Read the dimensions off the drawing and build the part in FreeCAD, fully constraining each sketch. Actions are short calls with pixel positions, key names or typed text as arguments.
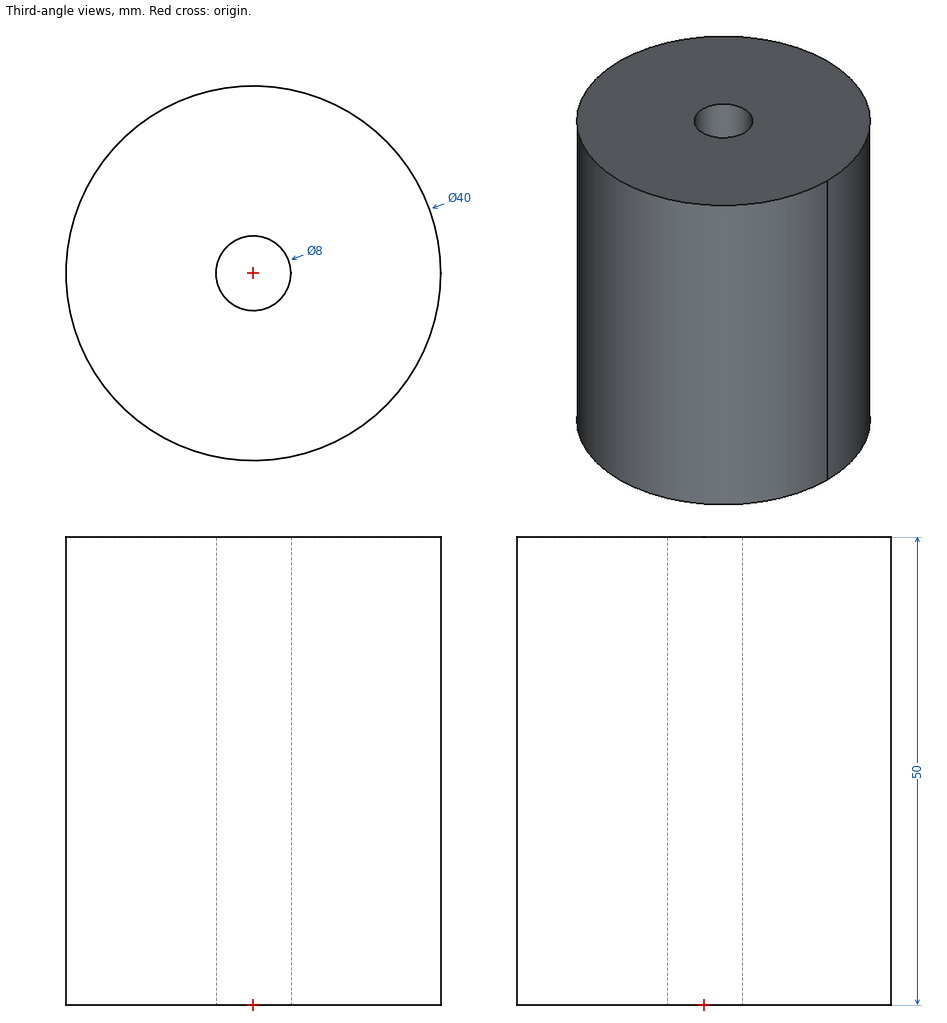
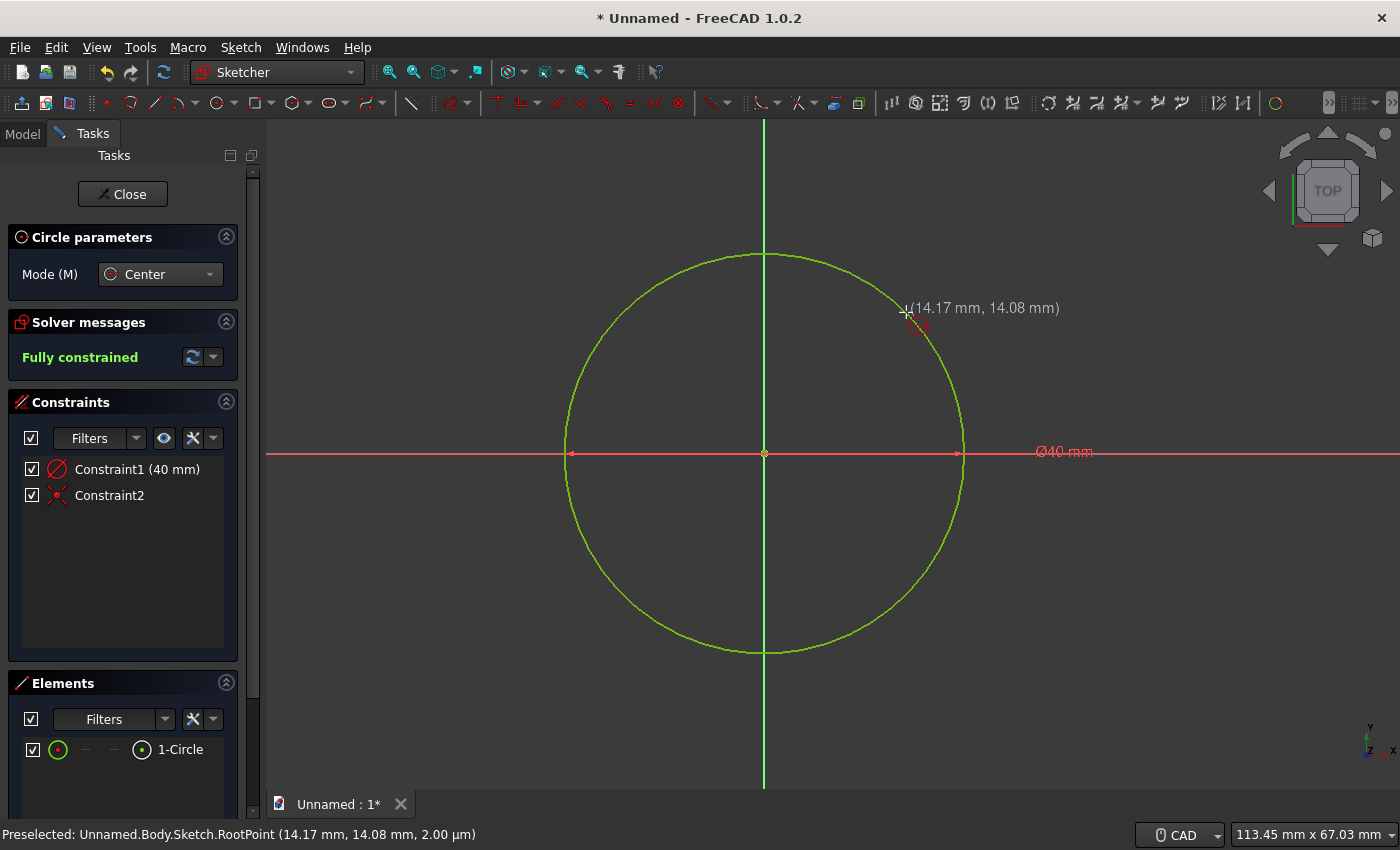
click(764, 454)
move(793, 425)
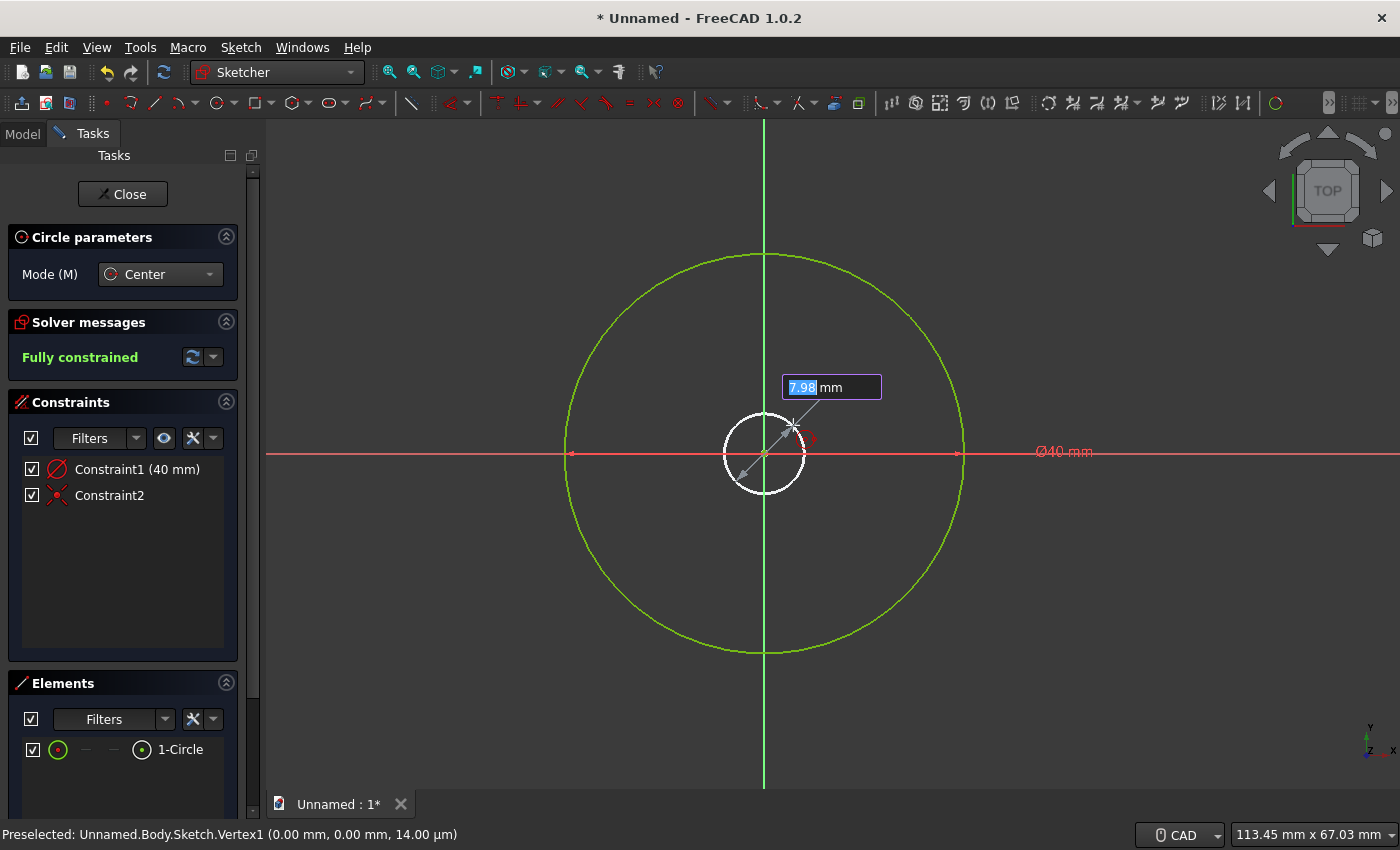
text(8)
key(Return)
key(Escape)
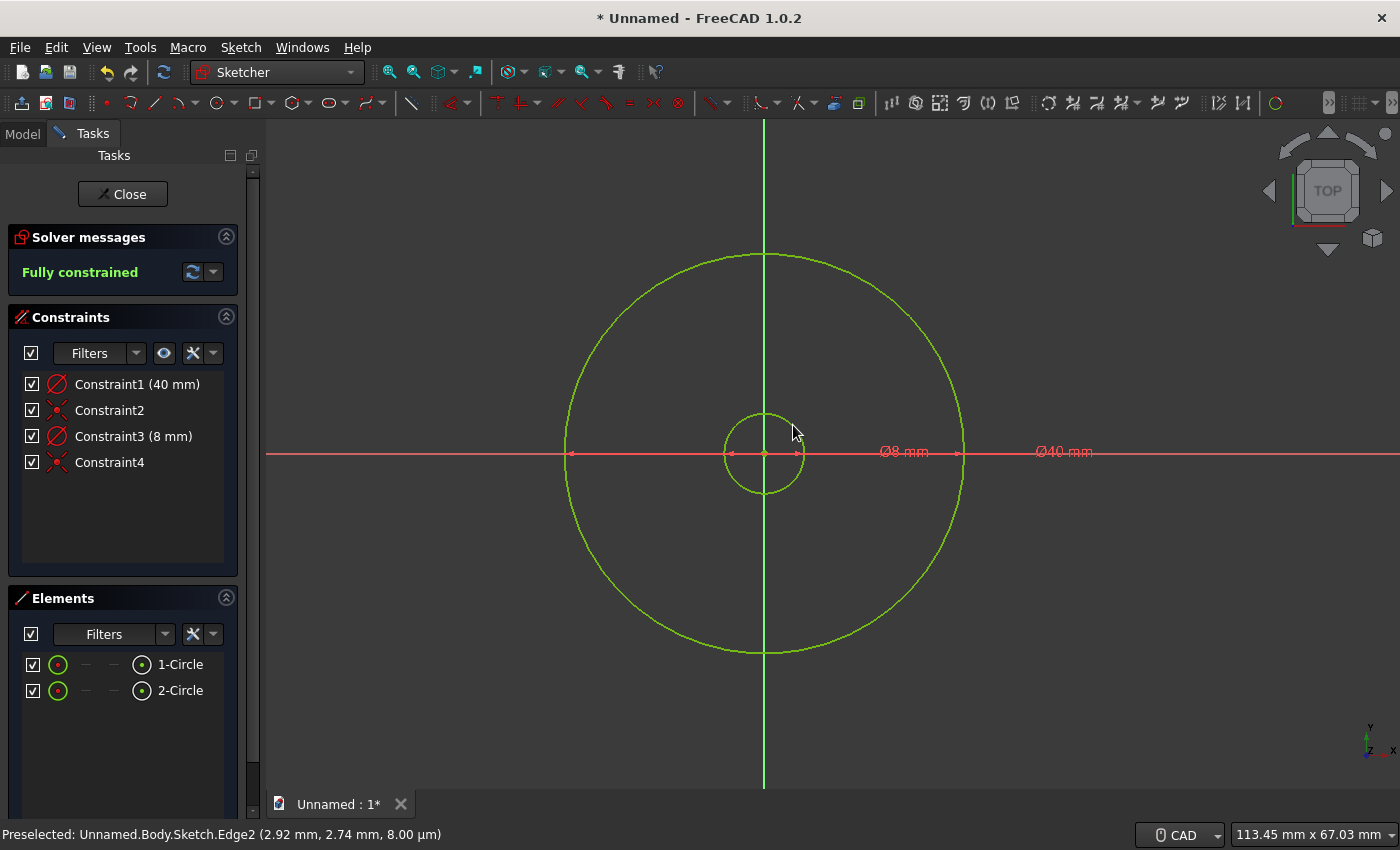
click(123, 194)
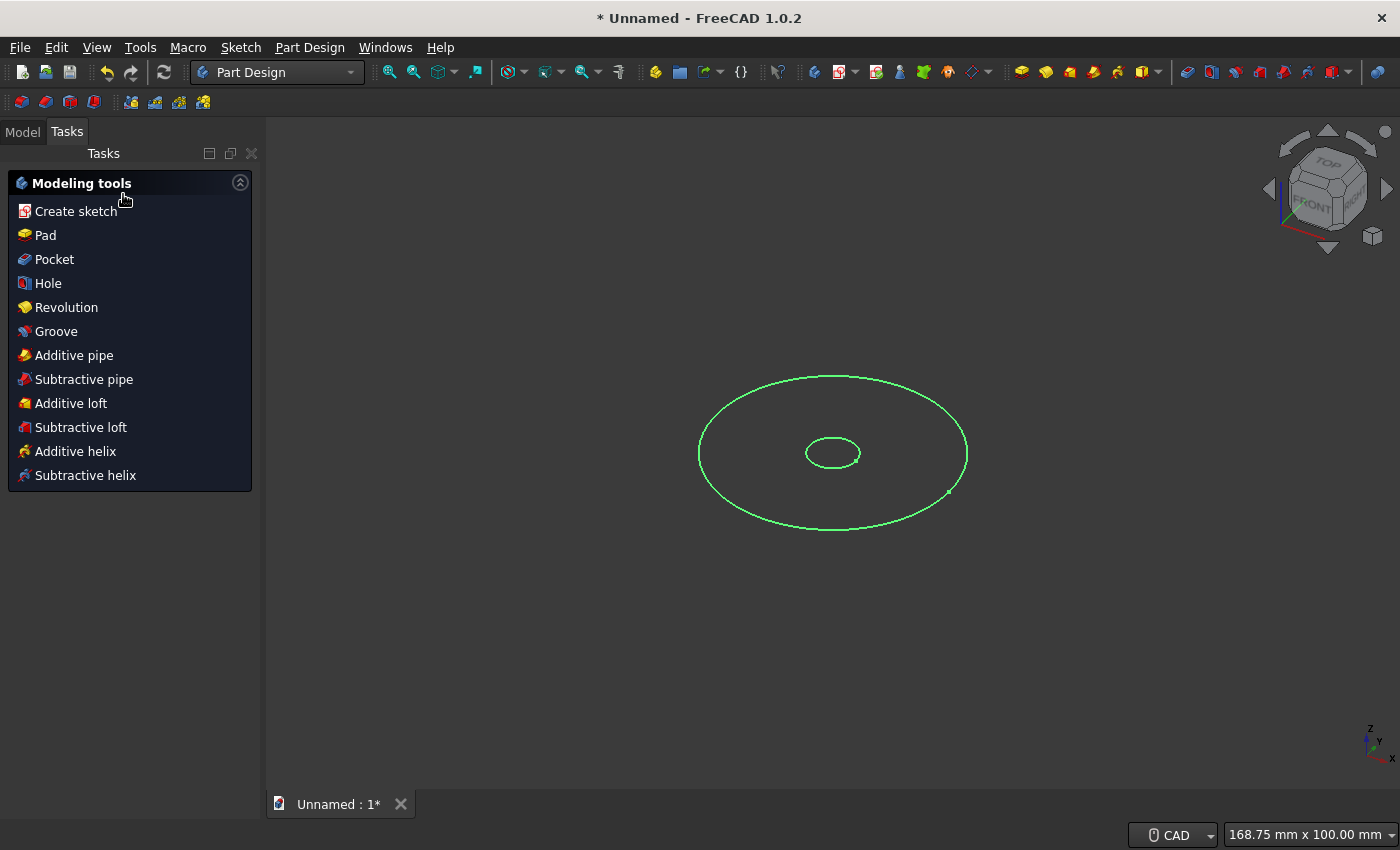
click(1022, 72)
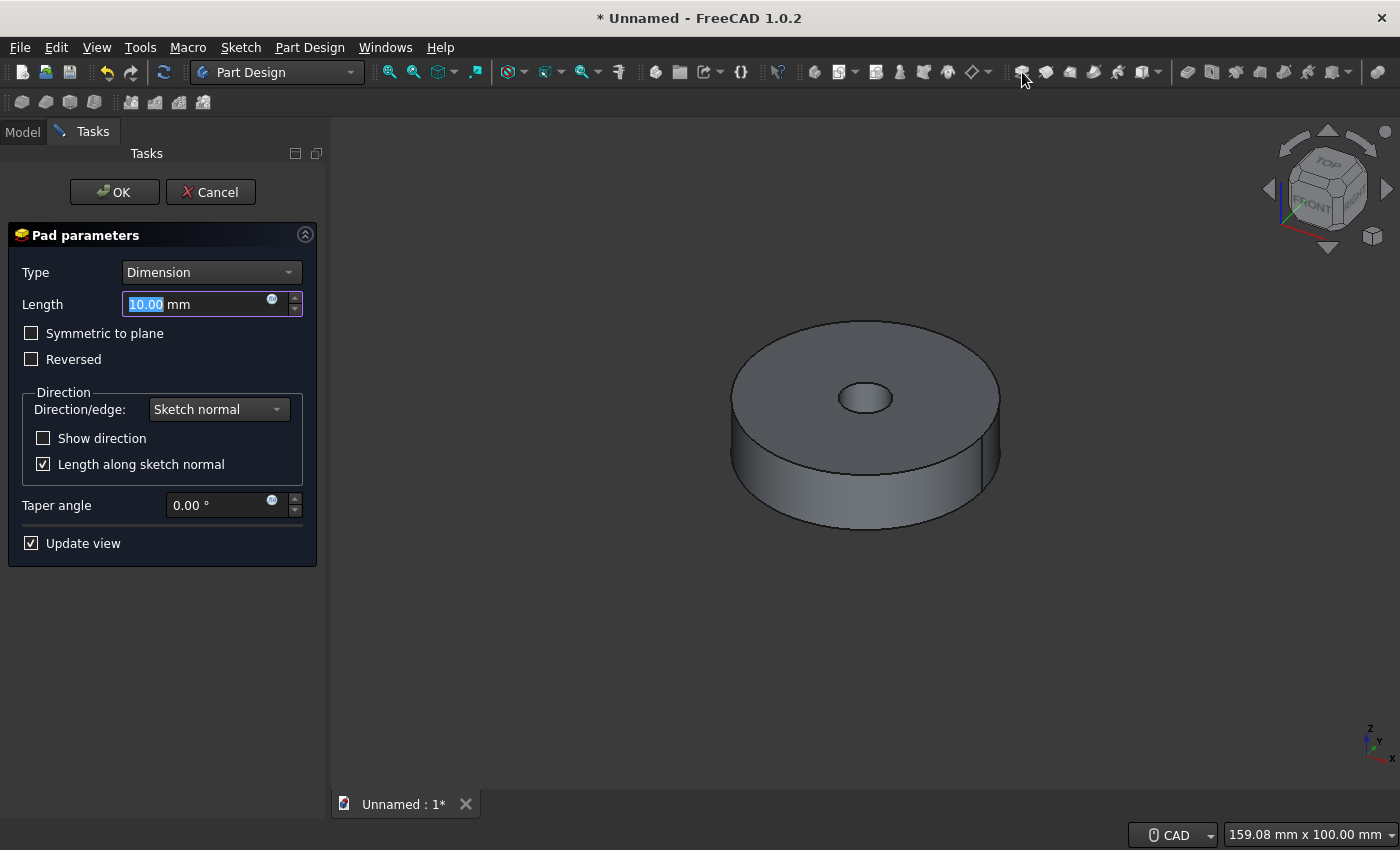
text(50)
key(Tab)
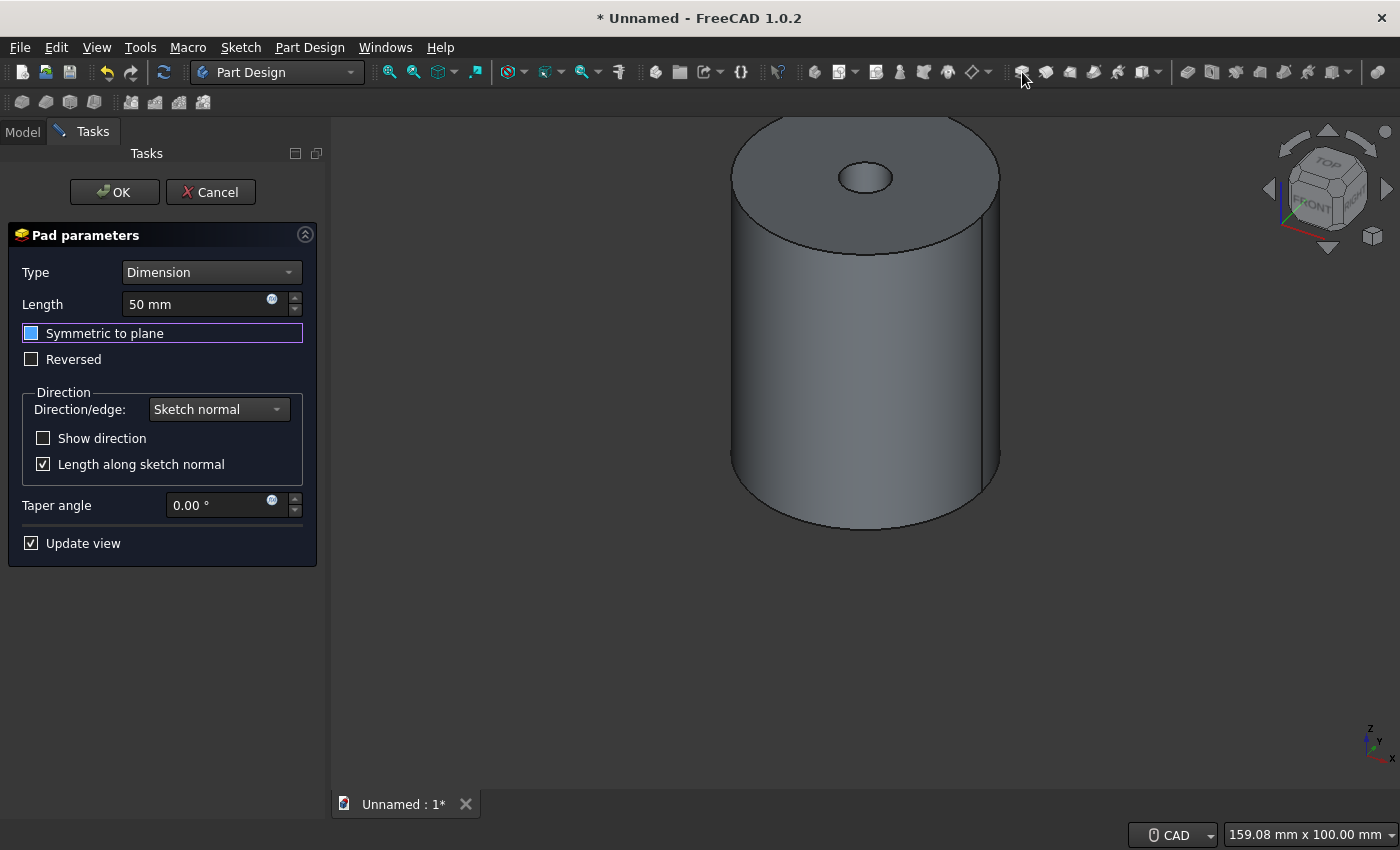
click(115, 192)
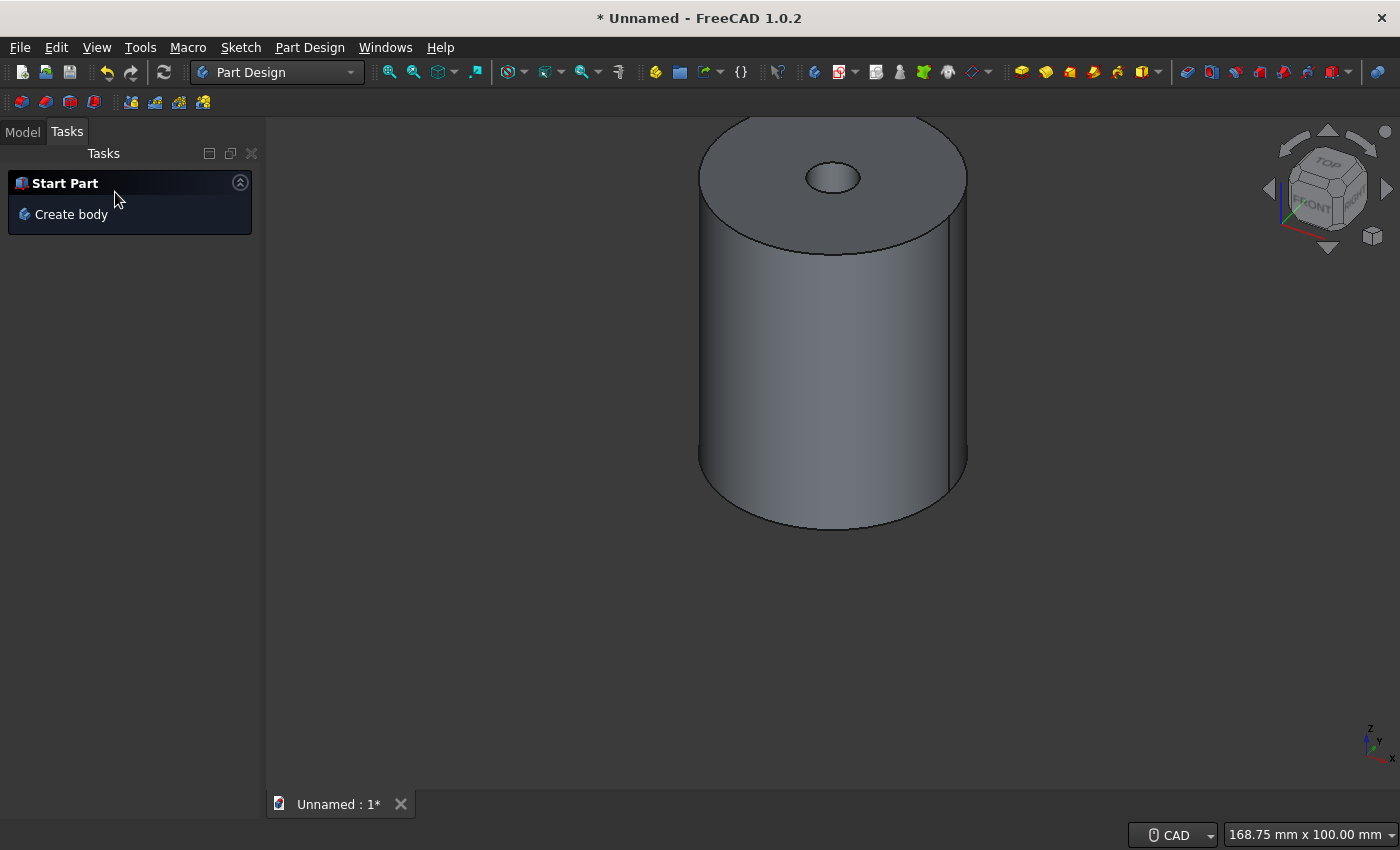
key(0)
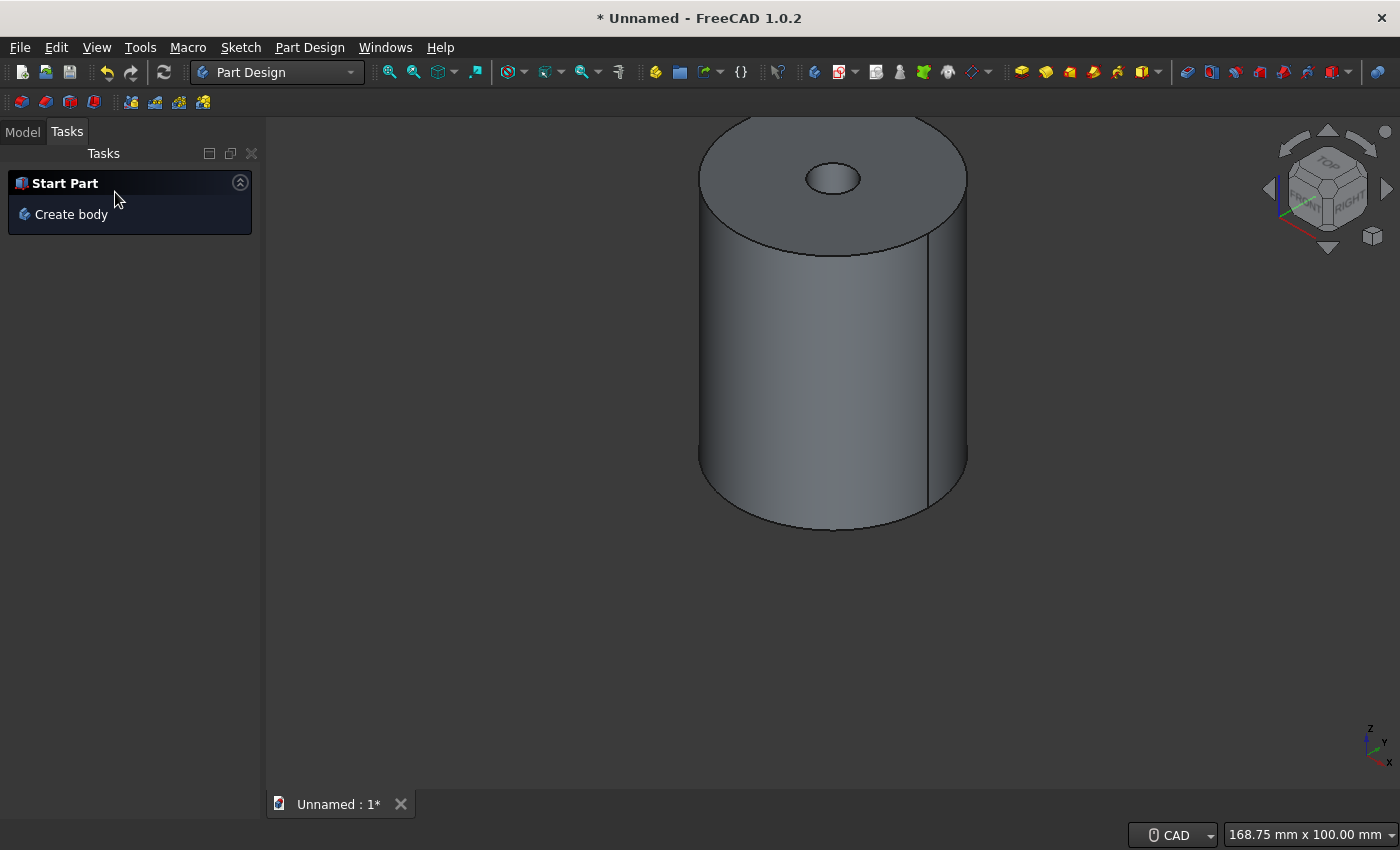
click(390, 72)